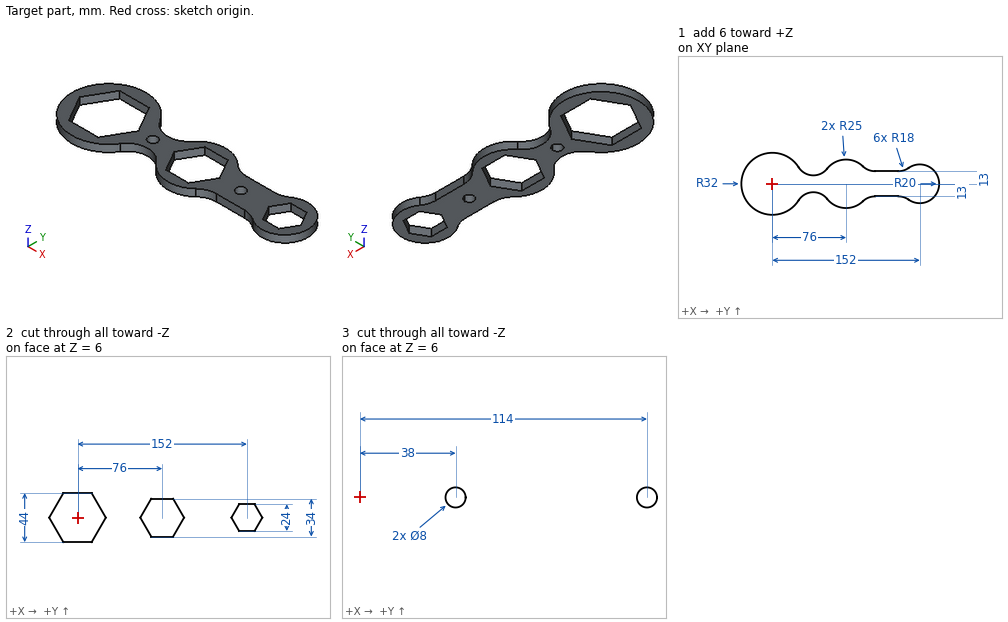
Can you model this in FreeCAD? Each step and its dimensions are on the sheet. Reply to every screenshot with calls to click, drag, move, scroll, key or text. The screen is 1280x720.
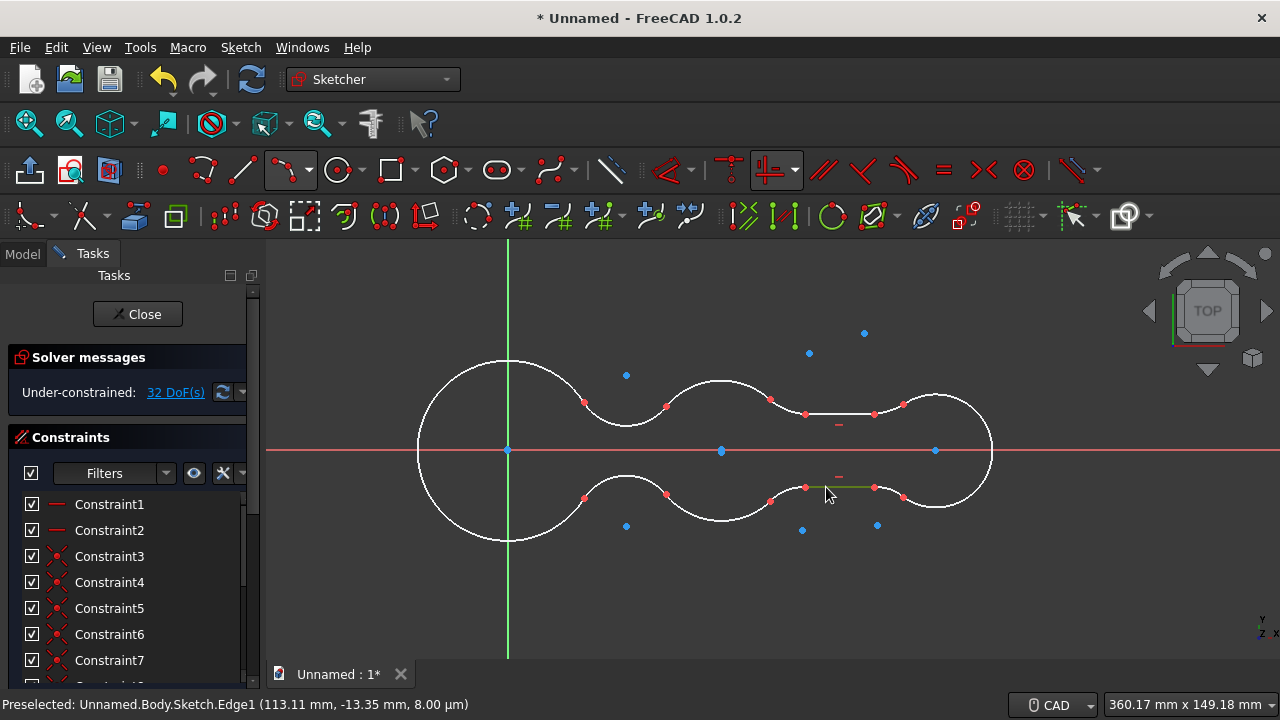
scroll(896, 492, up, 2)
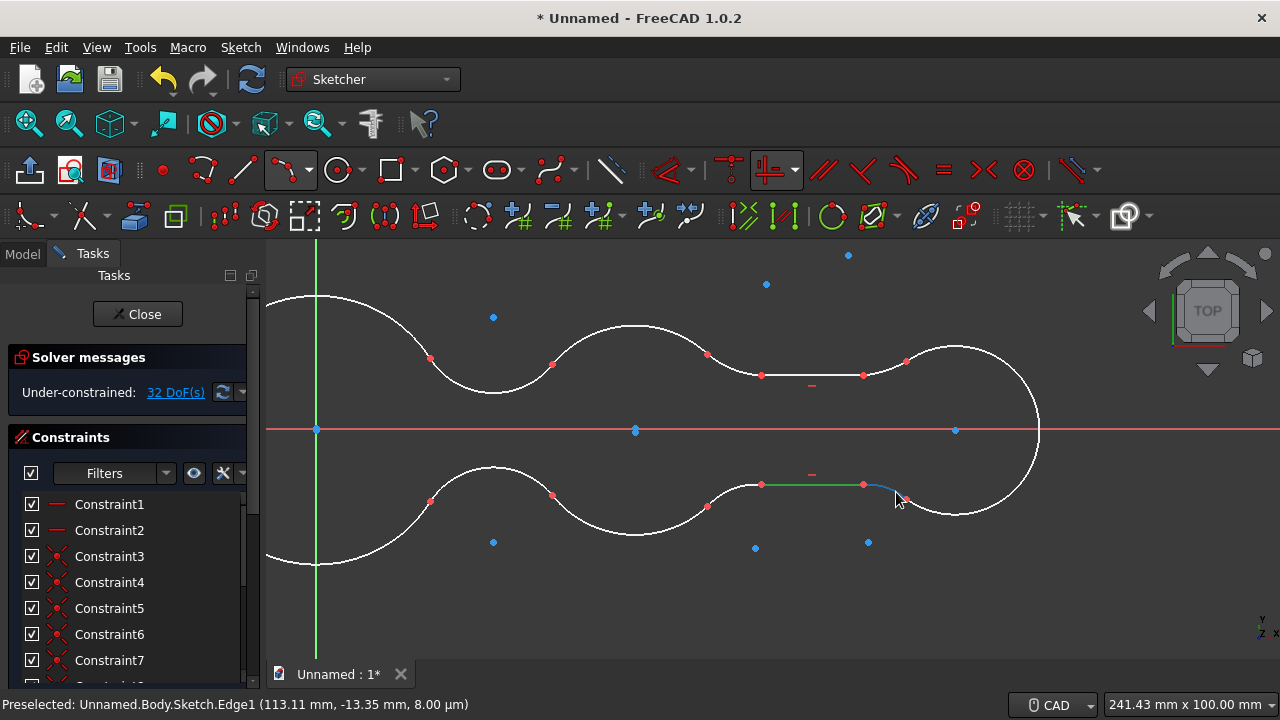
click(895, 491)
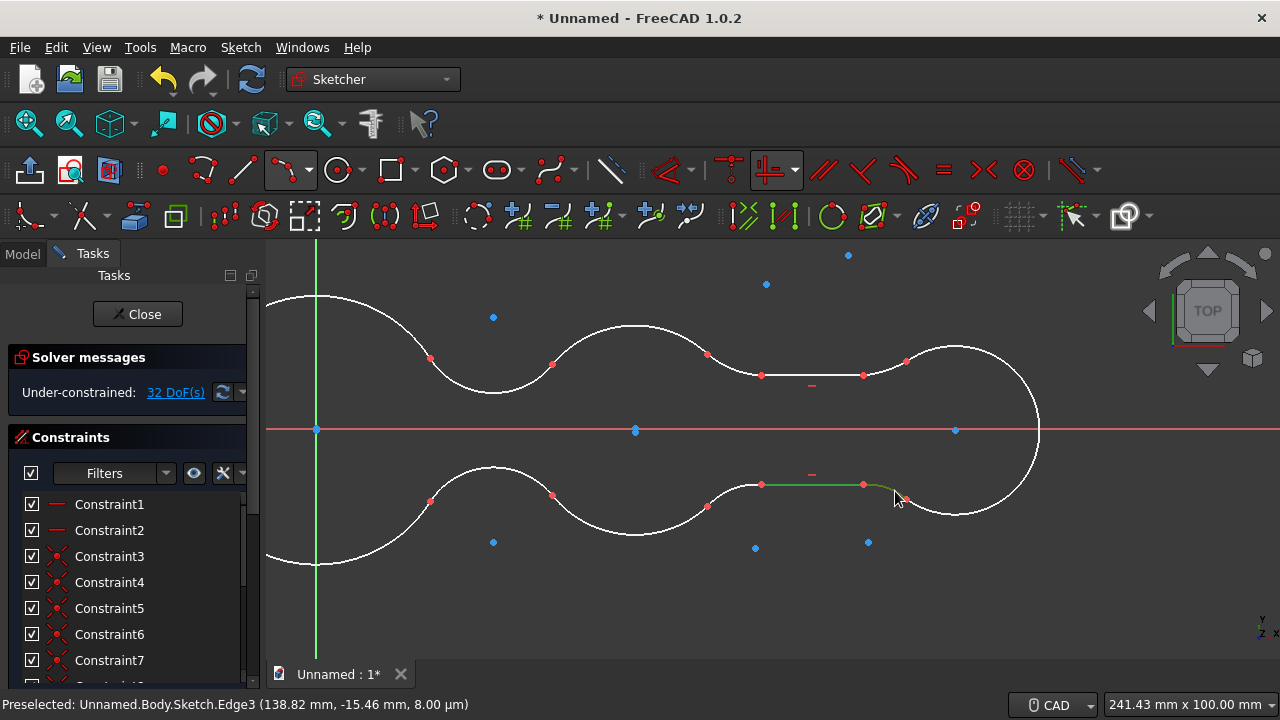
click(904, 170)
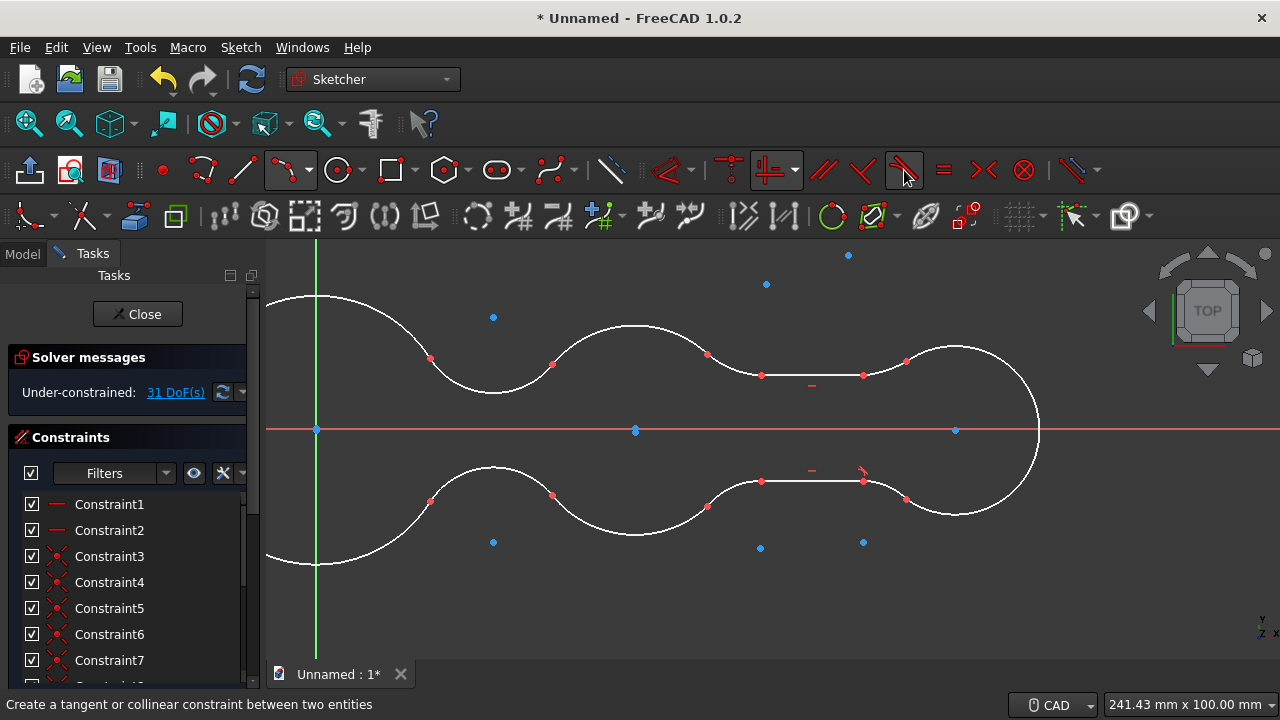
click(792, 481)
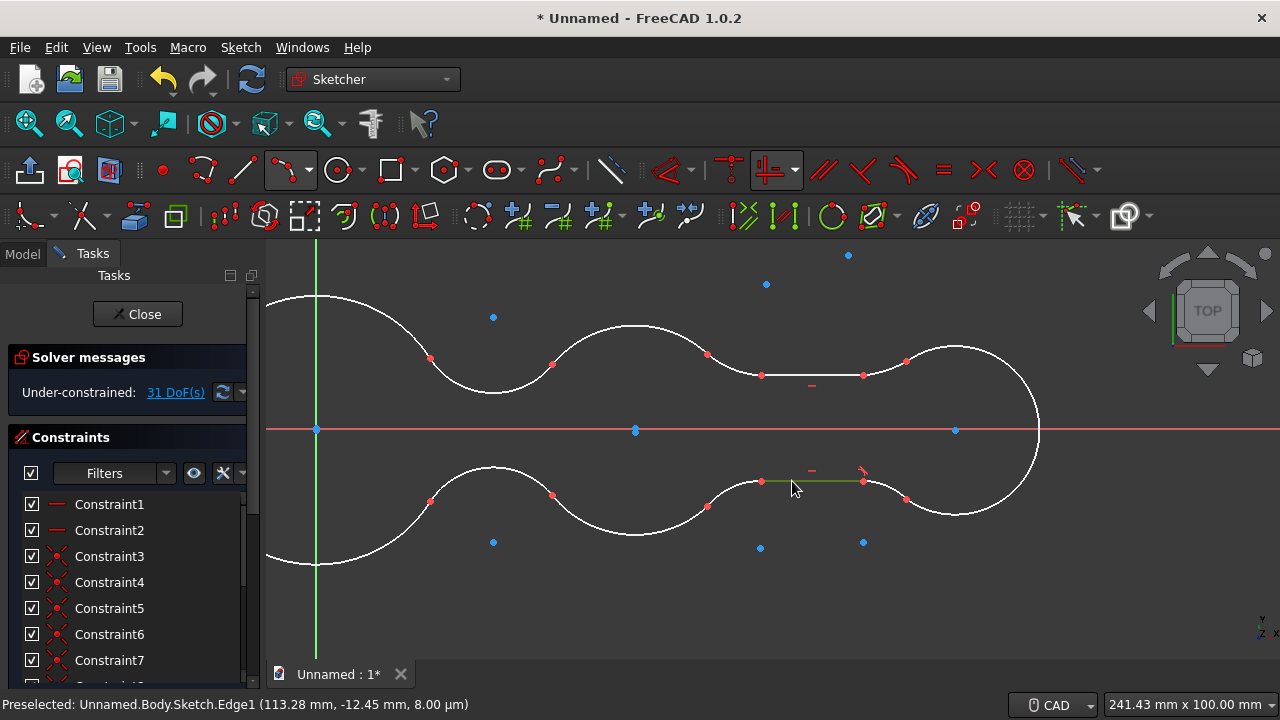
click(743, 483)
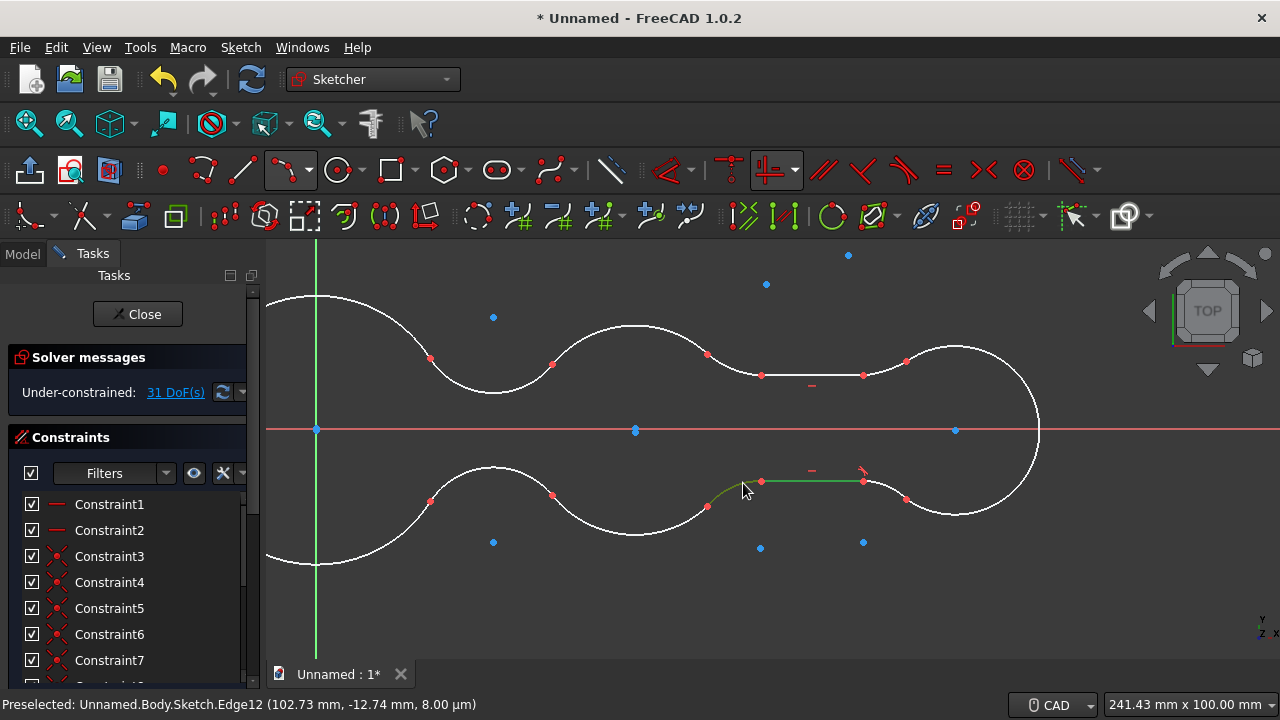
click(904, 170)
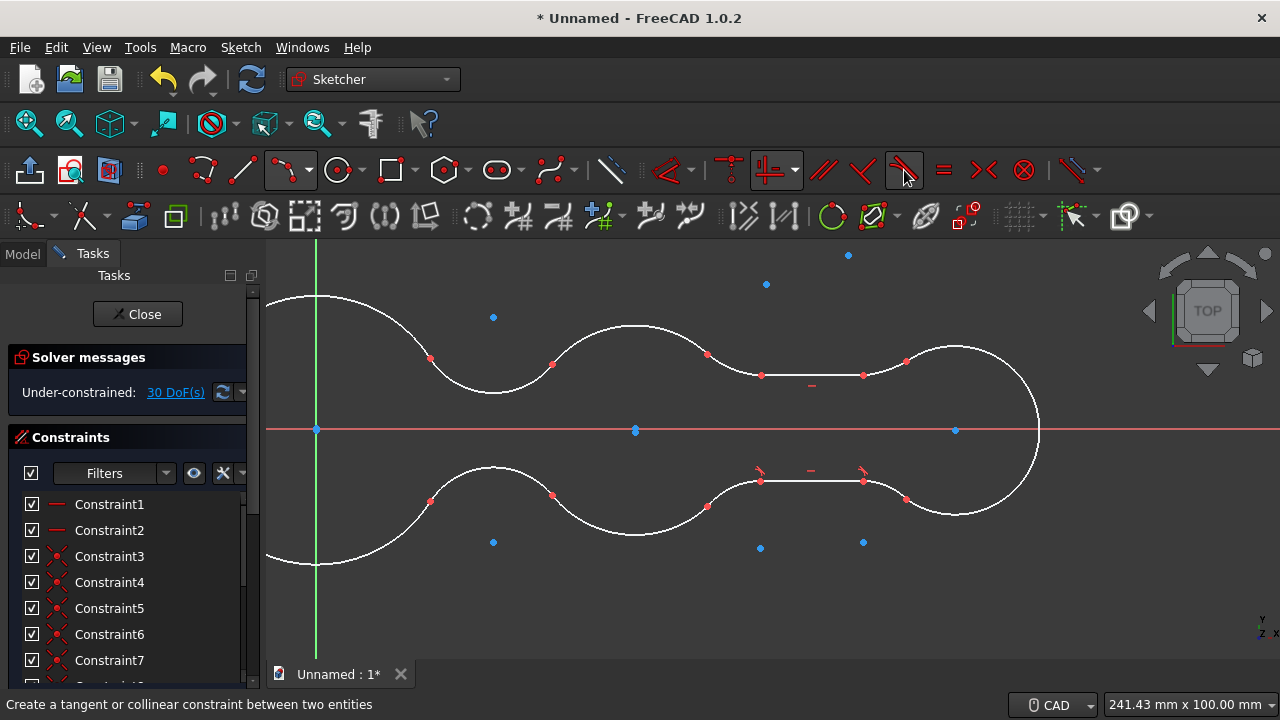
click(832, 375)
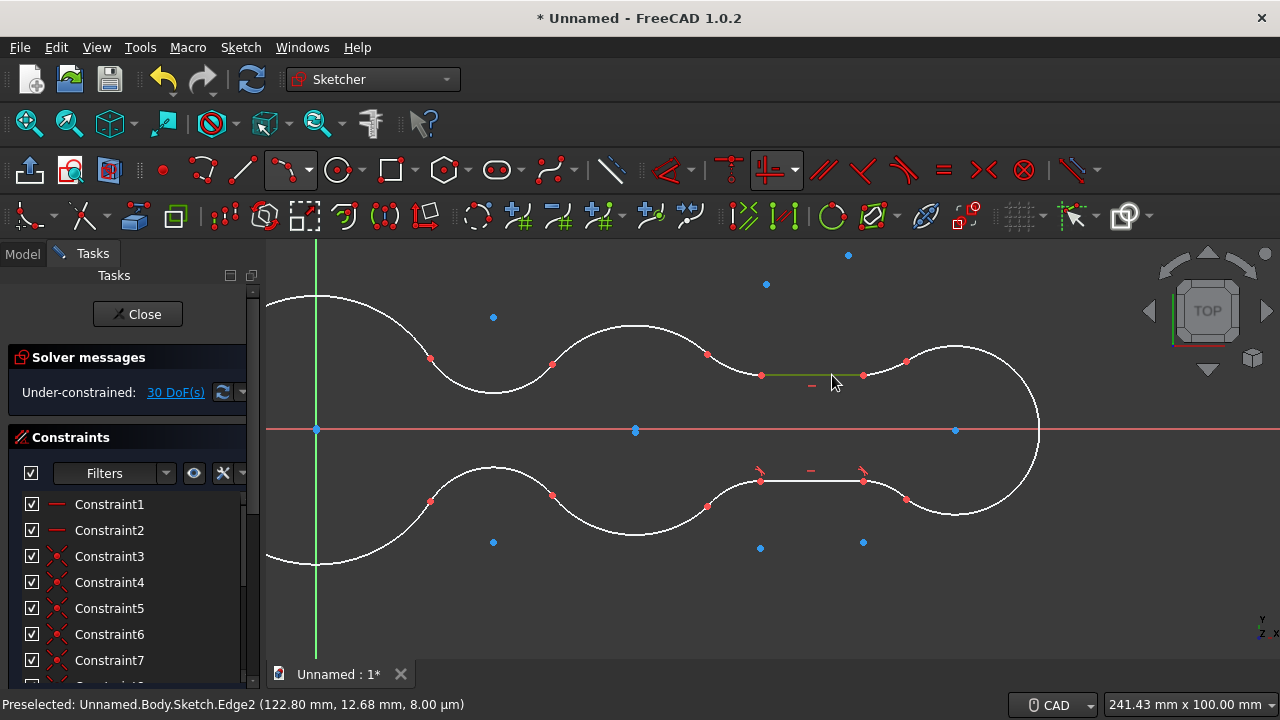
click(876, 373)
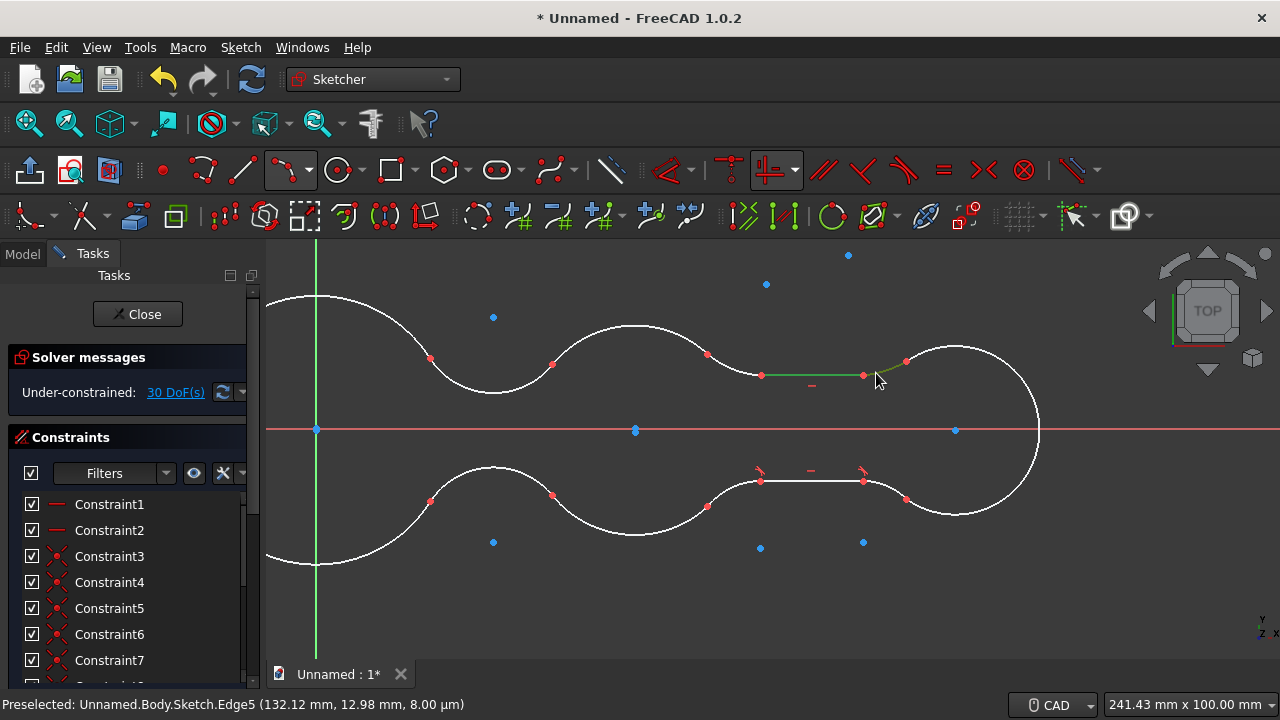
click(904, 170)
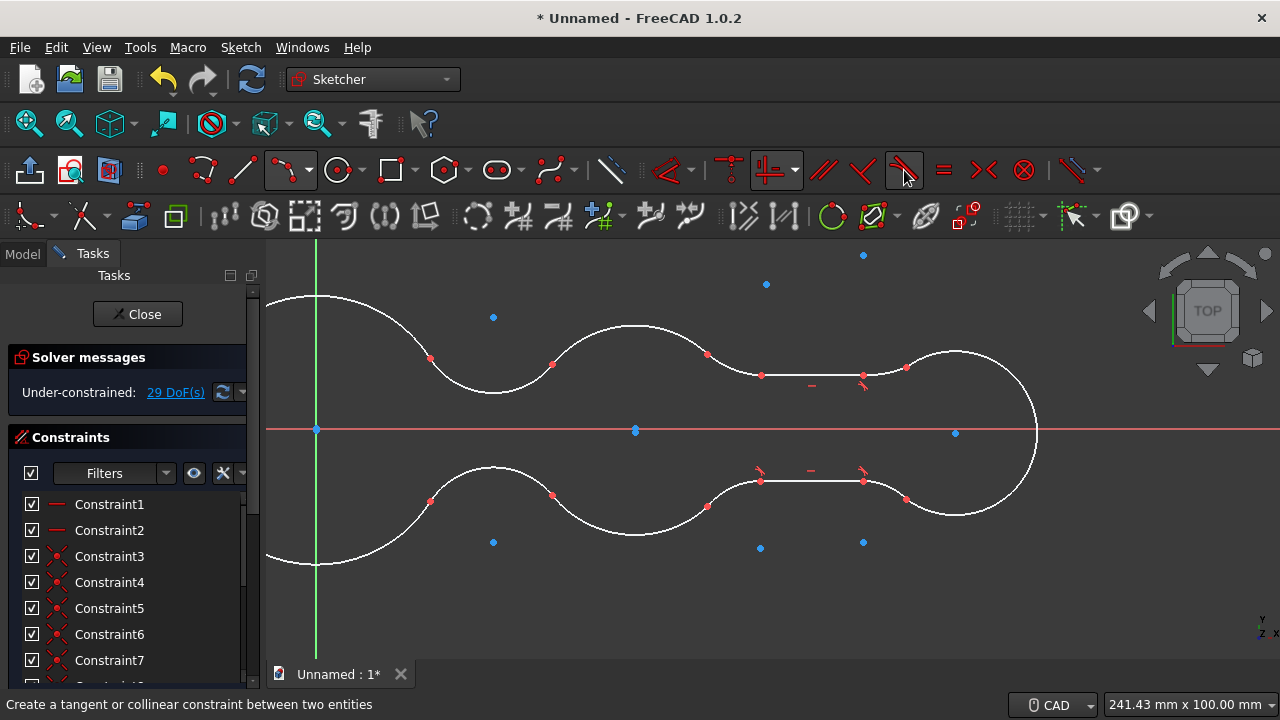
click(832, 375)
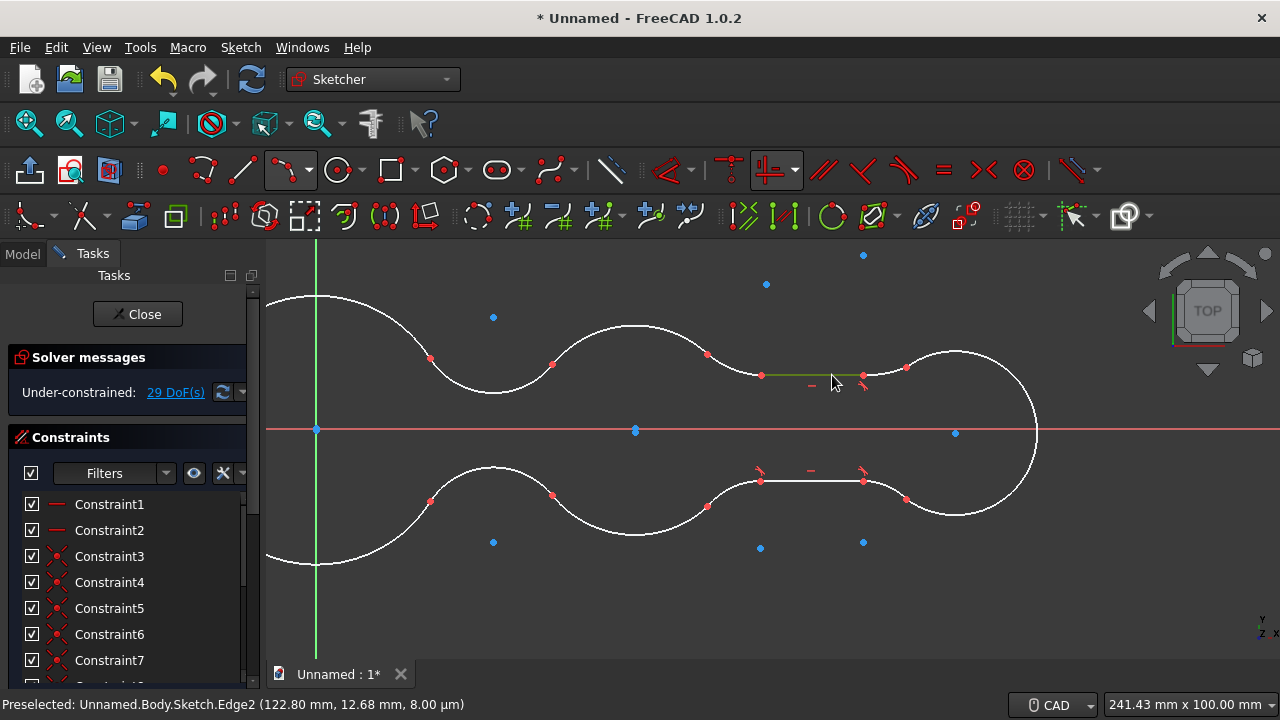
click(722, 364)